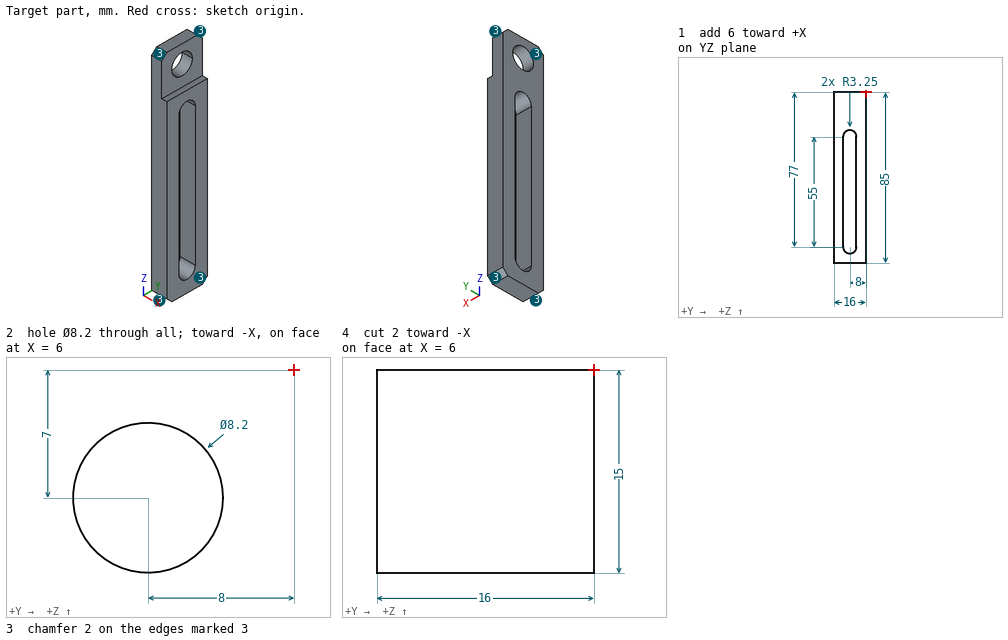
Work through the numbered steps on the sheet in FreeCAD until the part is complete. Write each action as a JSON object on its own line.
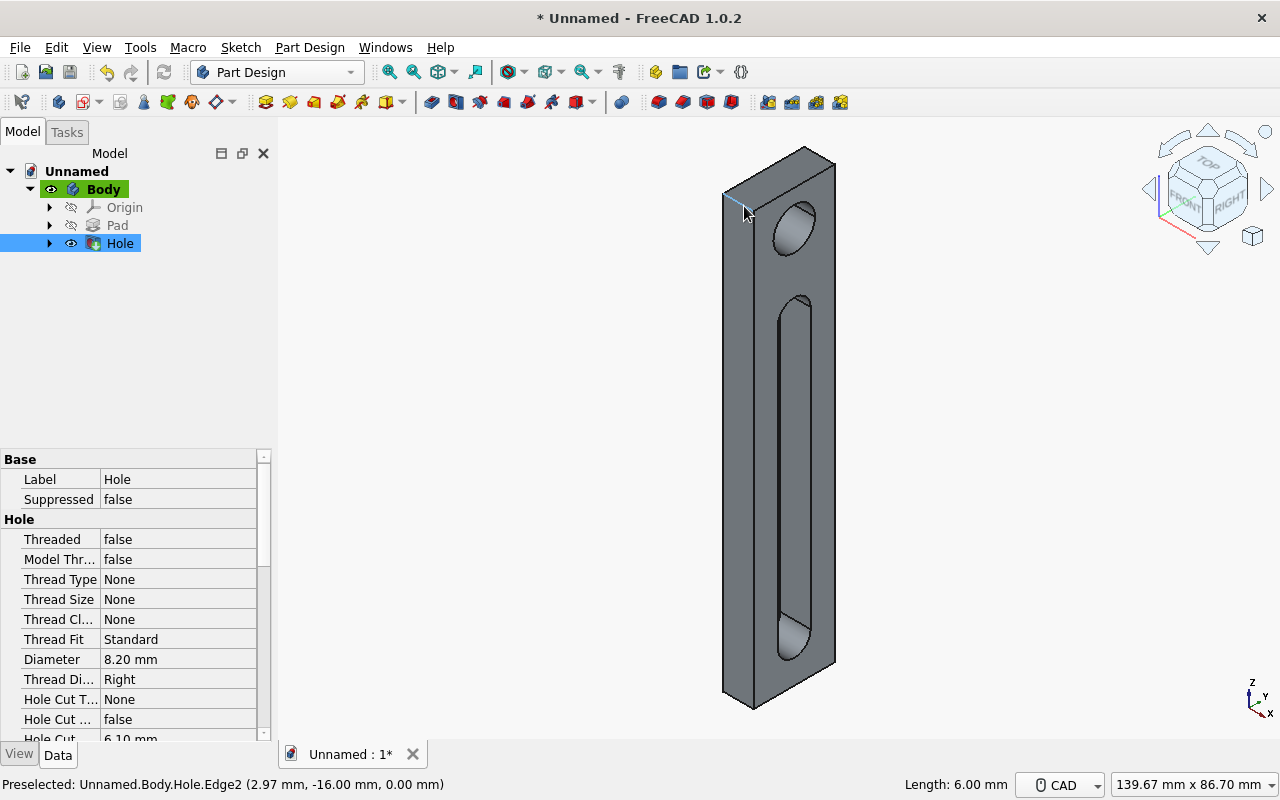
{"action": "key", "text": "2"}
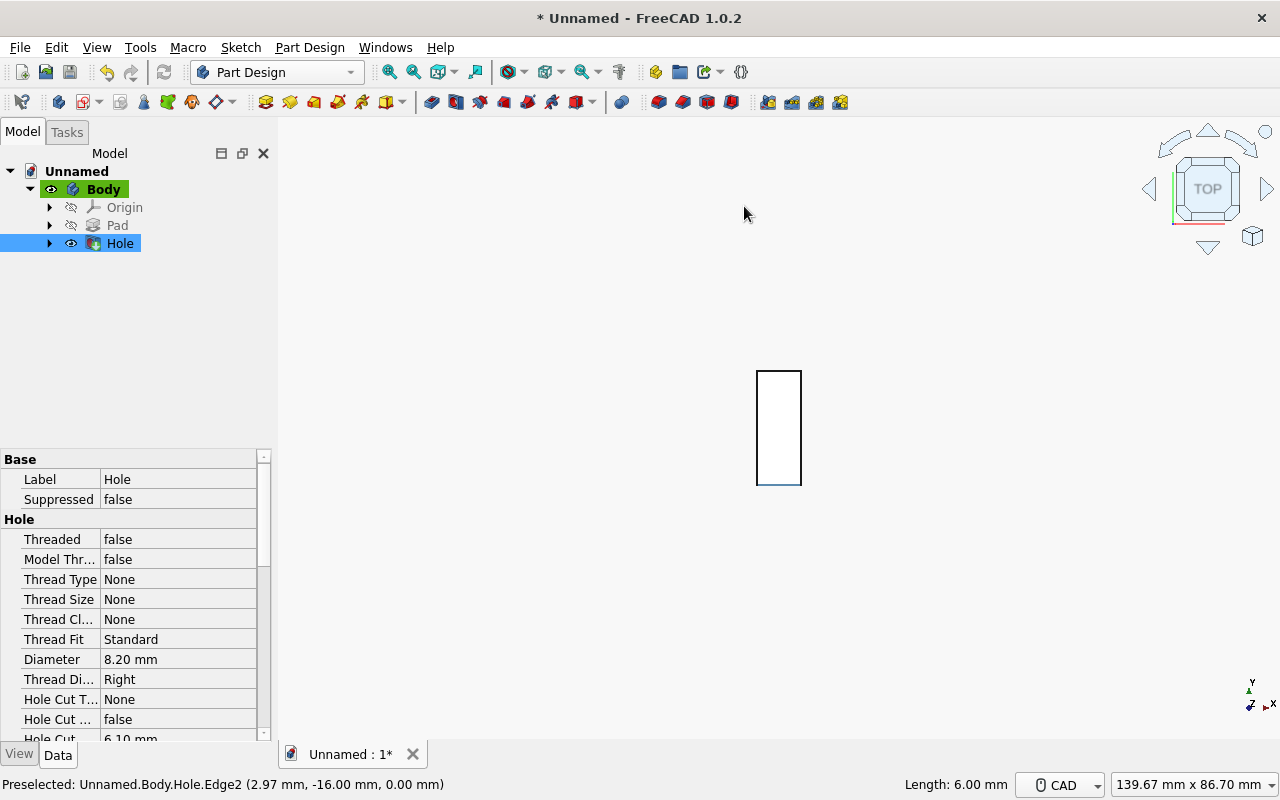
{"action": "left_click", "coordinate": [390, 72]}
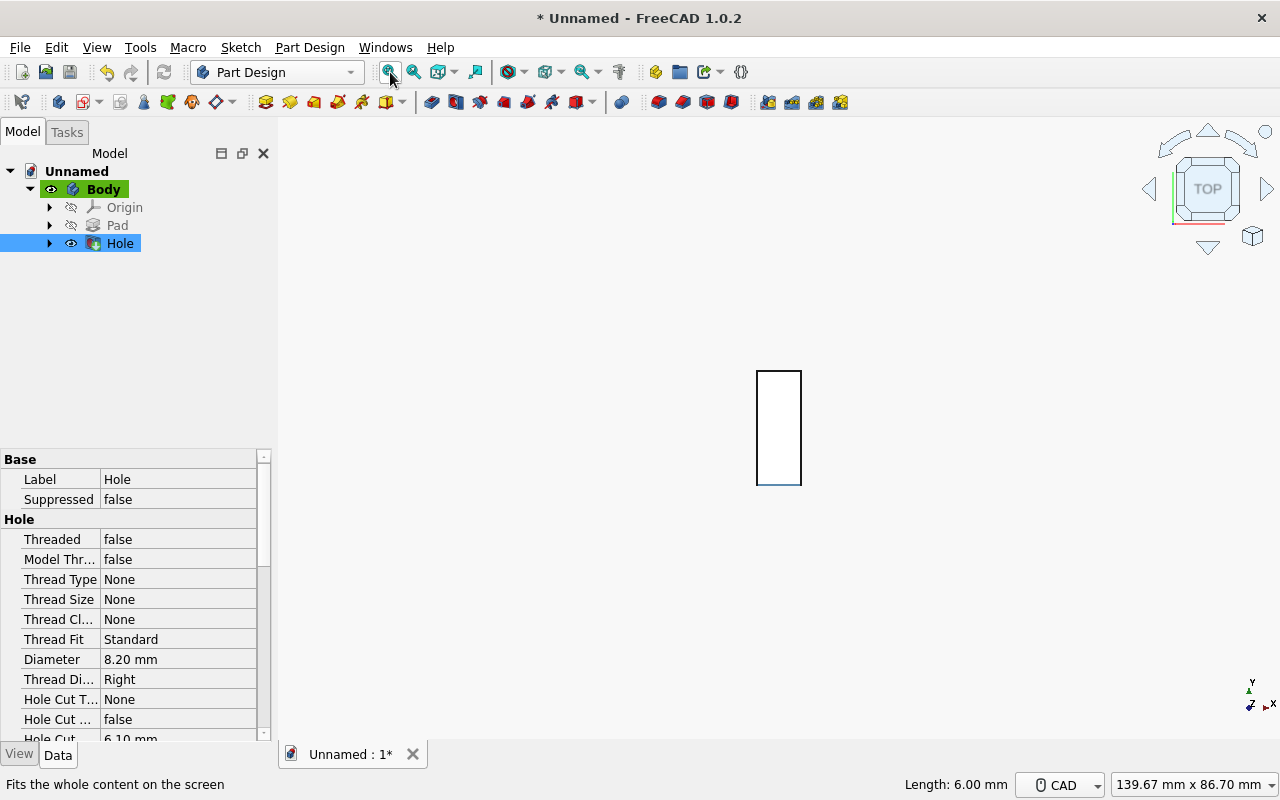
{"action": "key", "text": "1"}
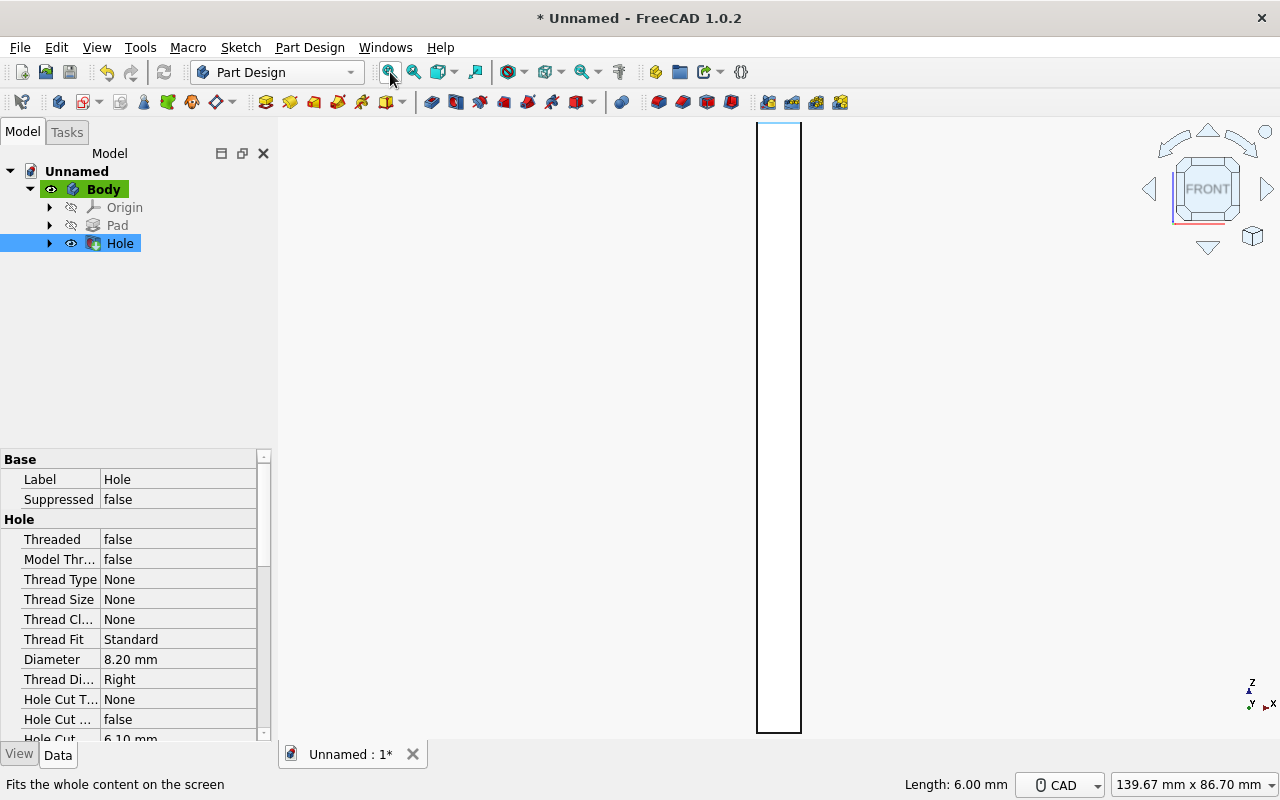
{"action": "key", "text": "3"}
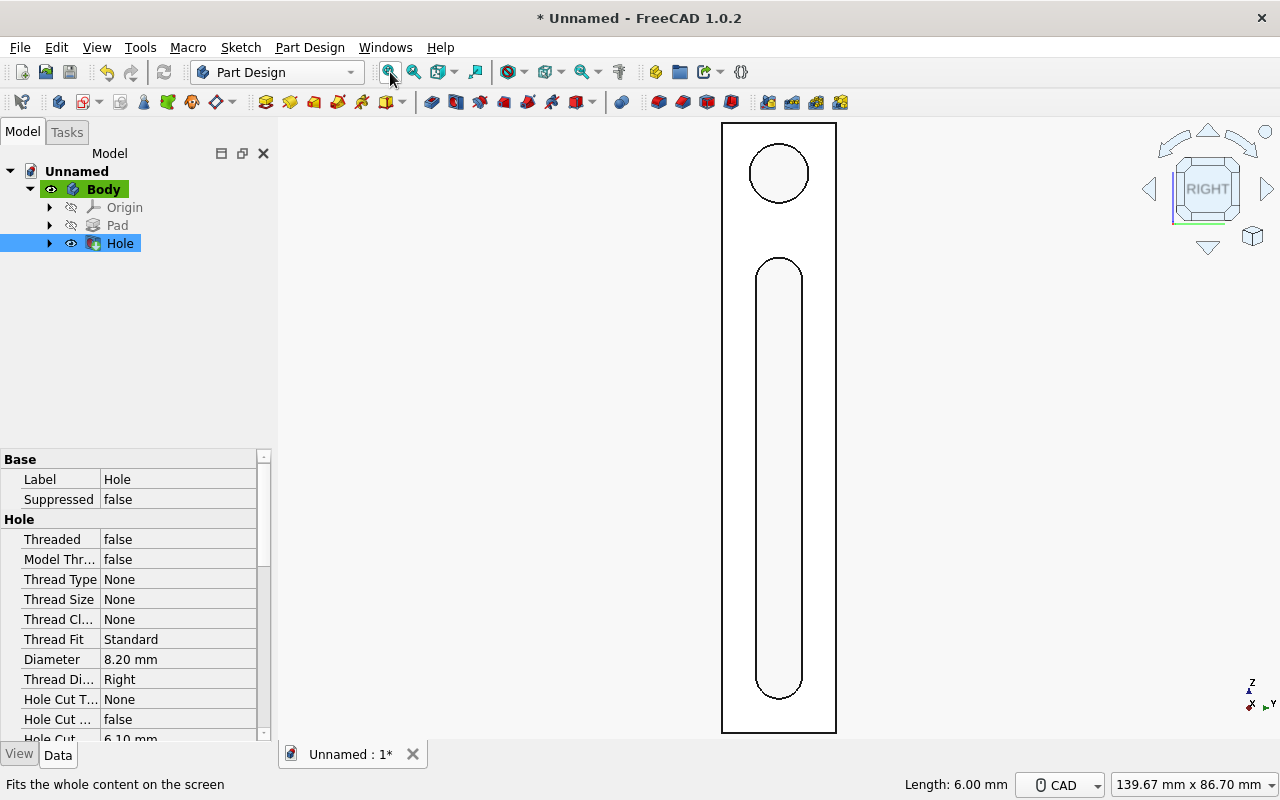
{"action": "key", "text": "5"}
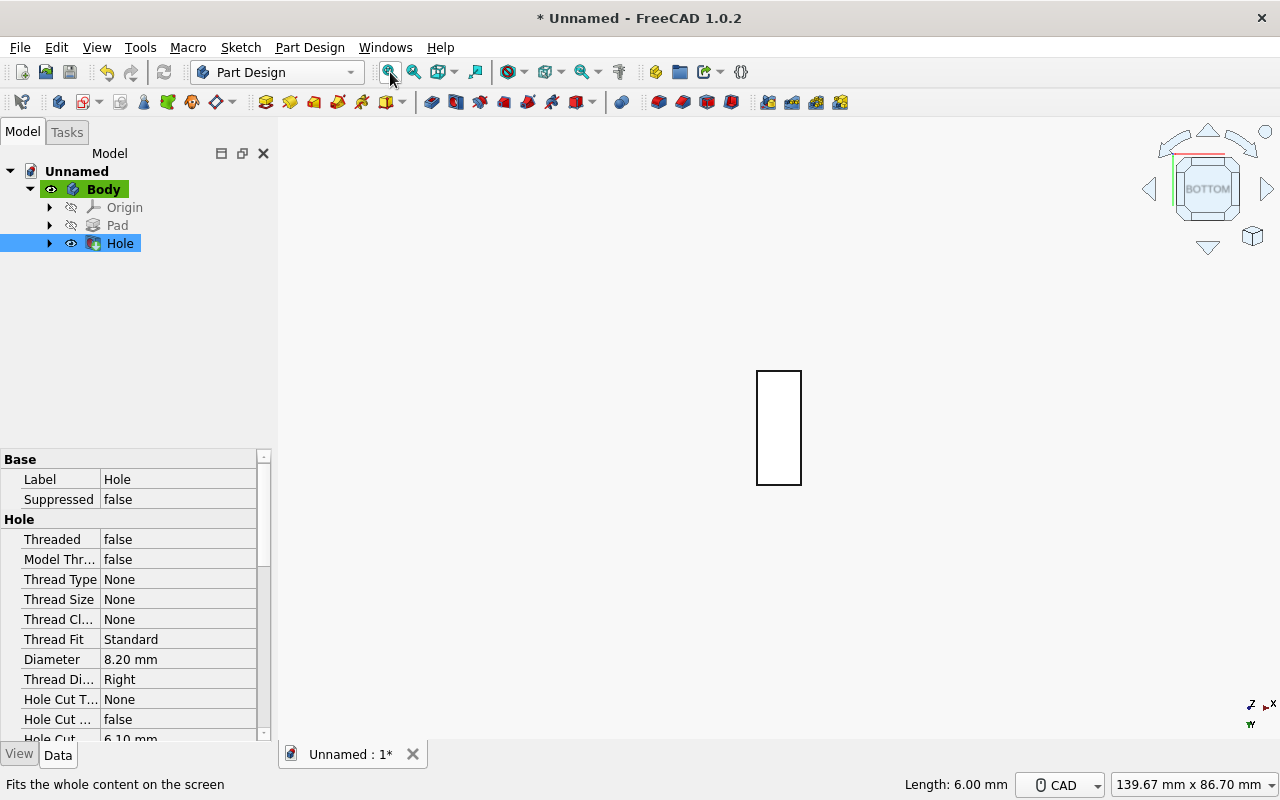
{"action": "left_click", "coordinate": [390, 72]}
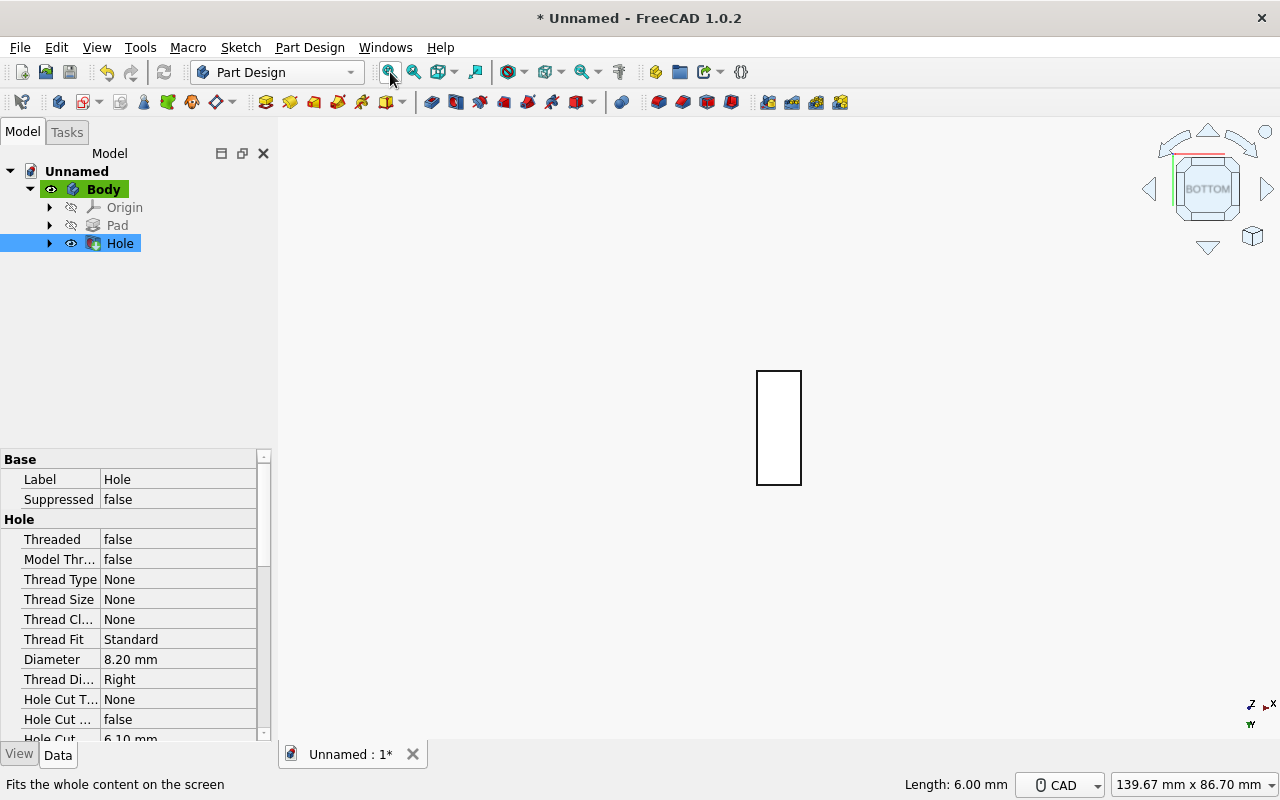
{"action": "left_click", "coordinate": [779, 484], "text": "ctrl"}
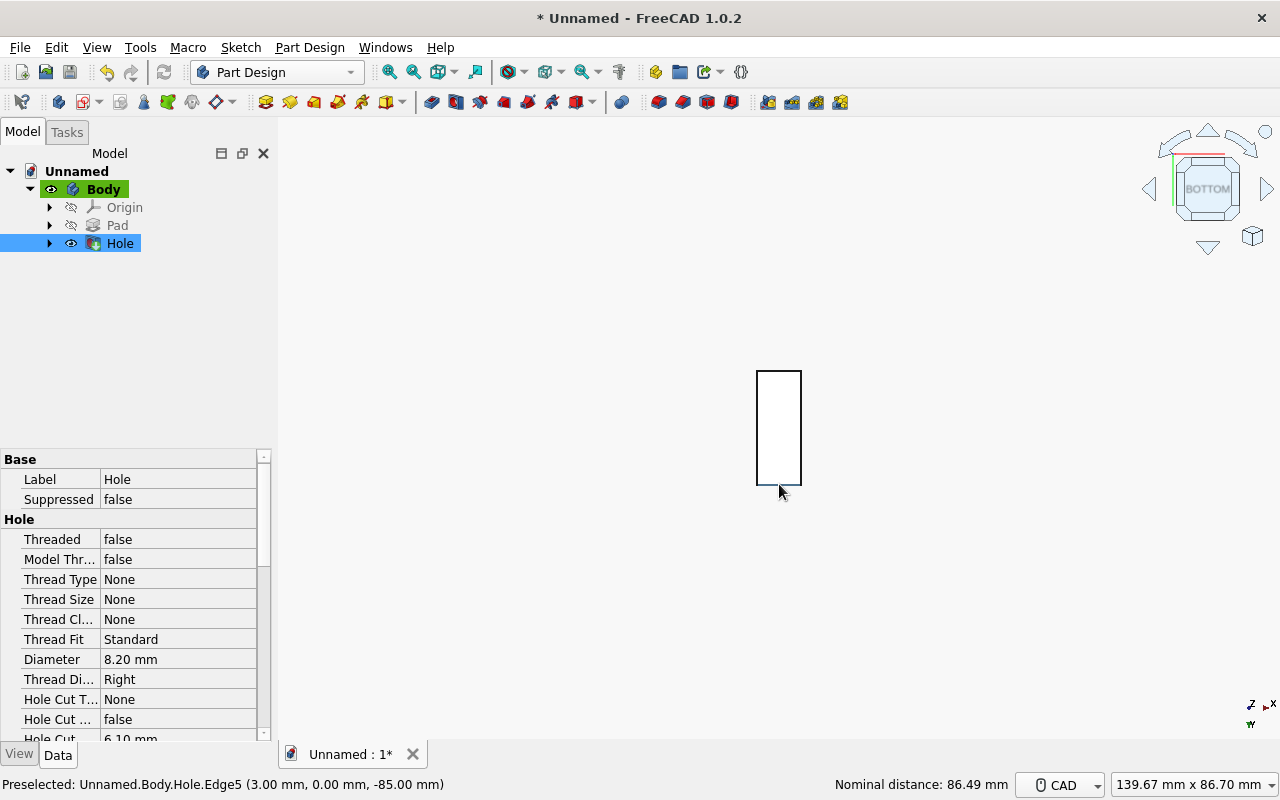
{"action": "left_click", "coordinate": [779, 370], "text": "ctrl"}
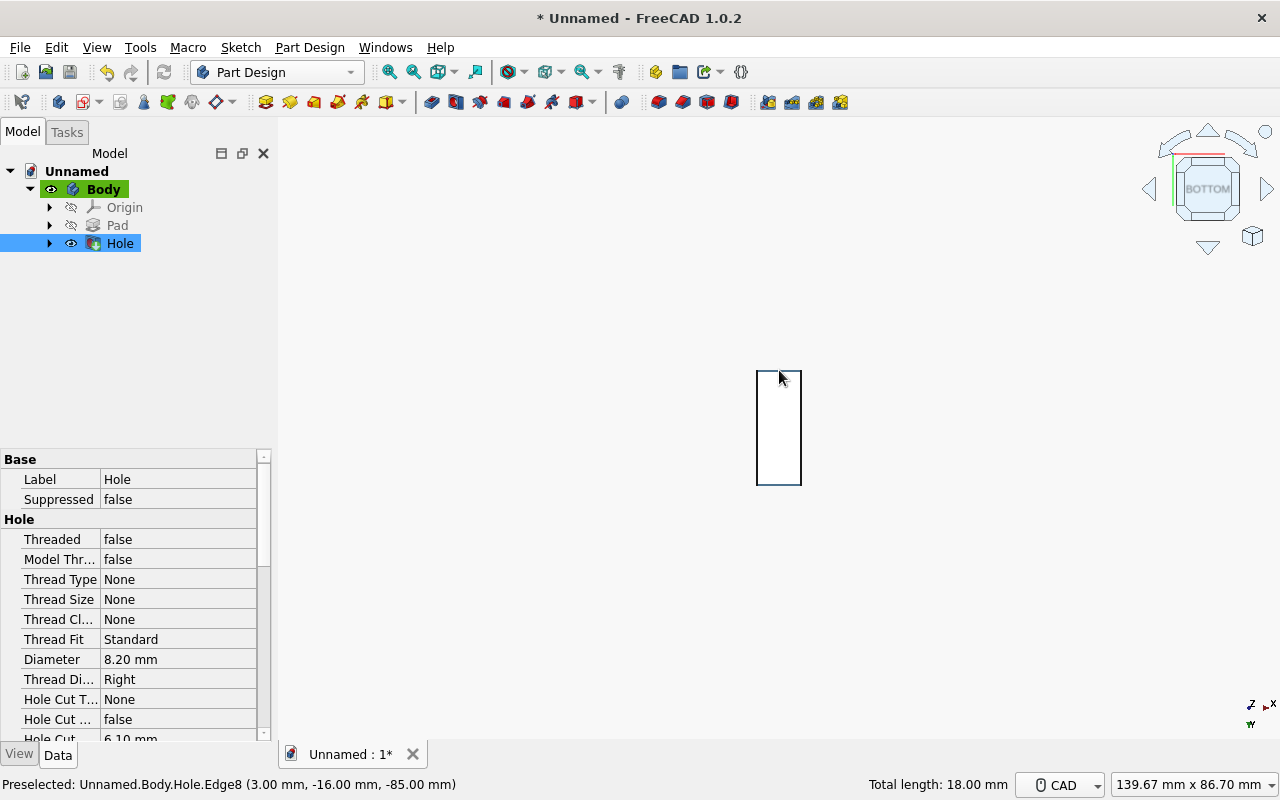
{"action": "key", "text": "4"}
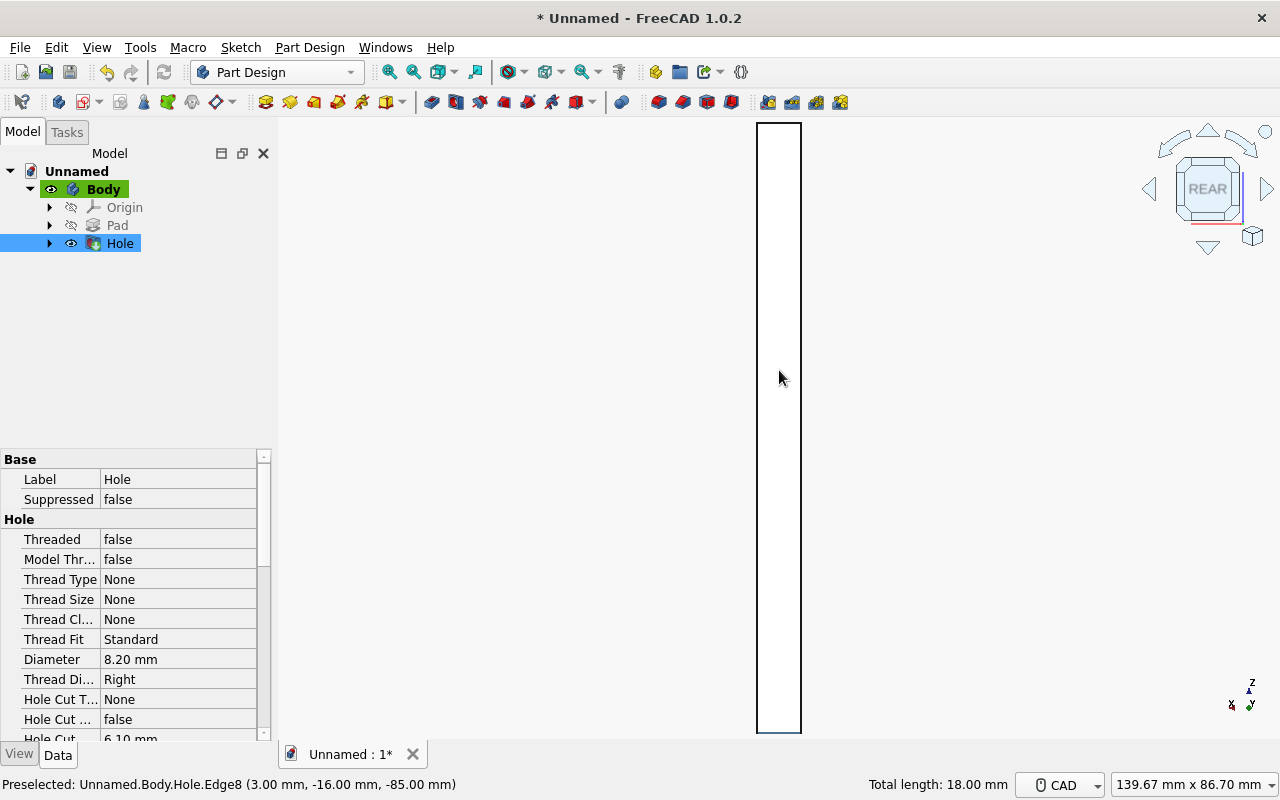
{"action": "key", "text": "6"}